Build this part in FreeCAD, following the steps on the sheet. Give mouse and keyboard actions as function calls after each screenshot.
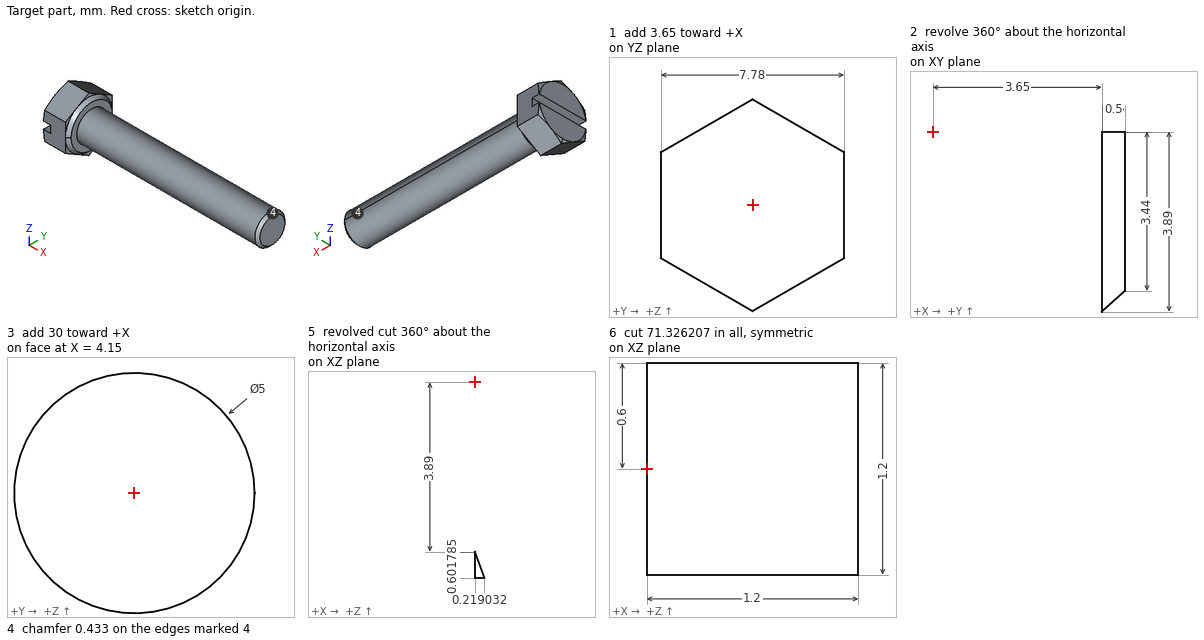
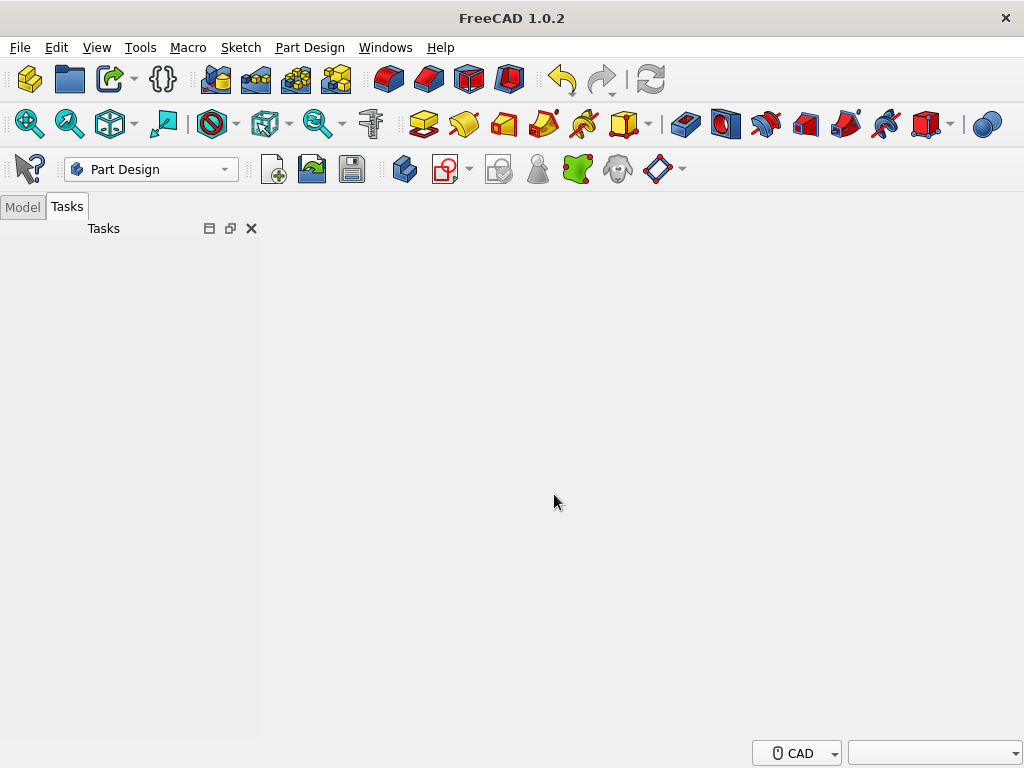
key(ctrl+n)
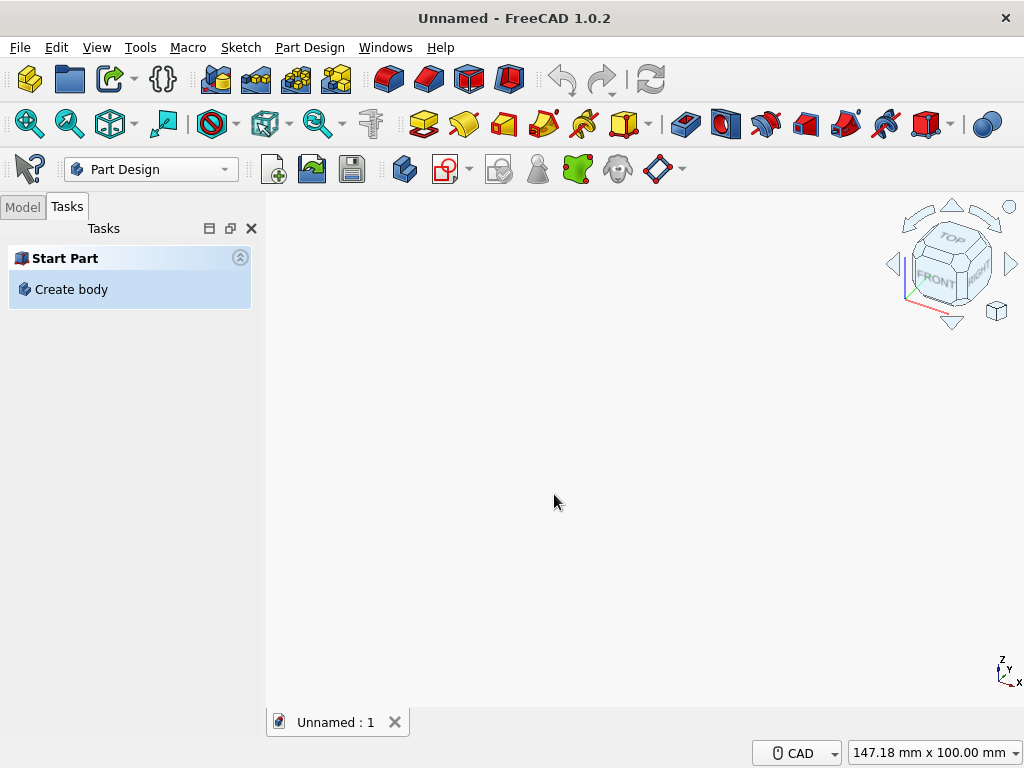
click(446, 170)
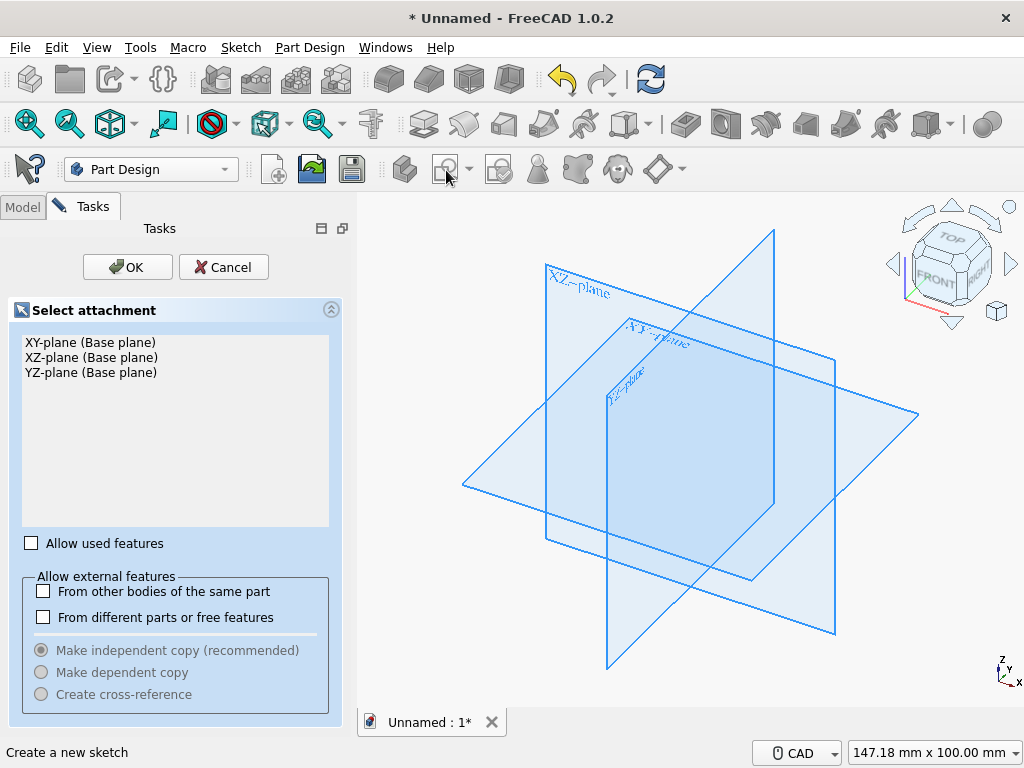
click(82, 372)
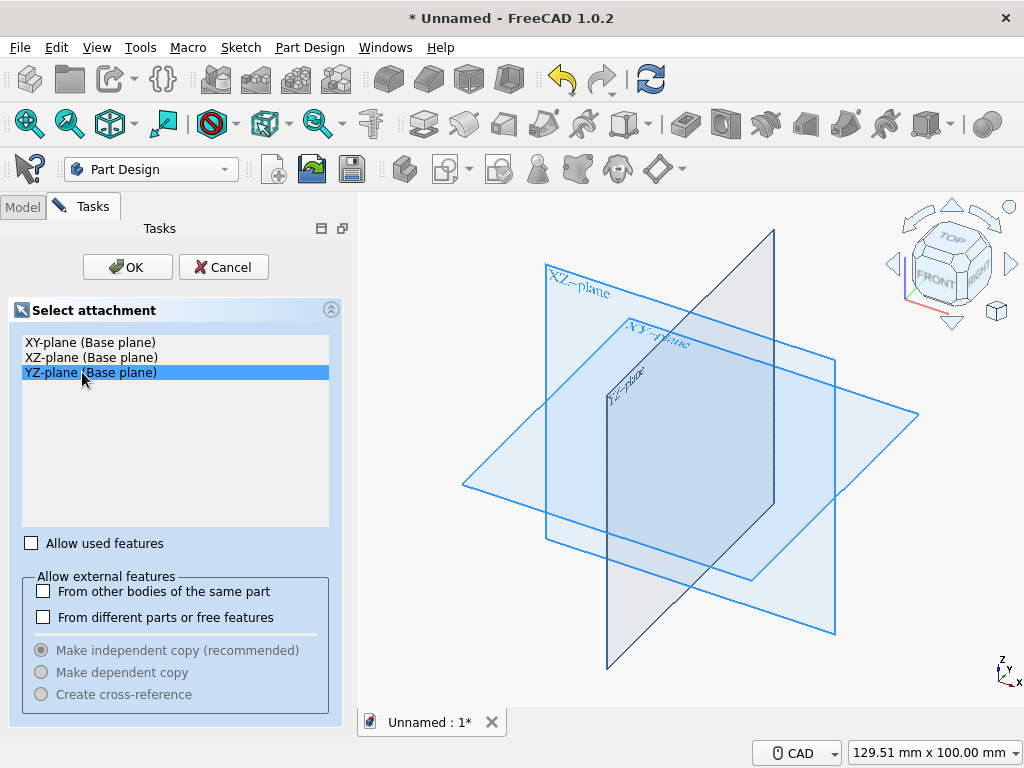
click(128, 267)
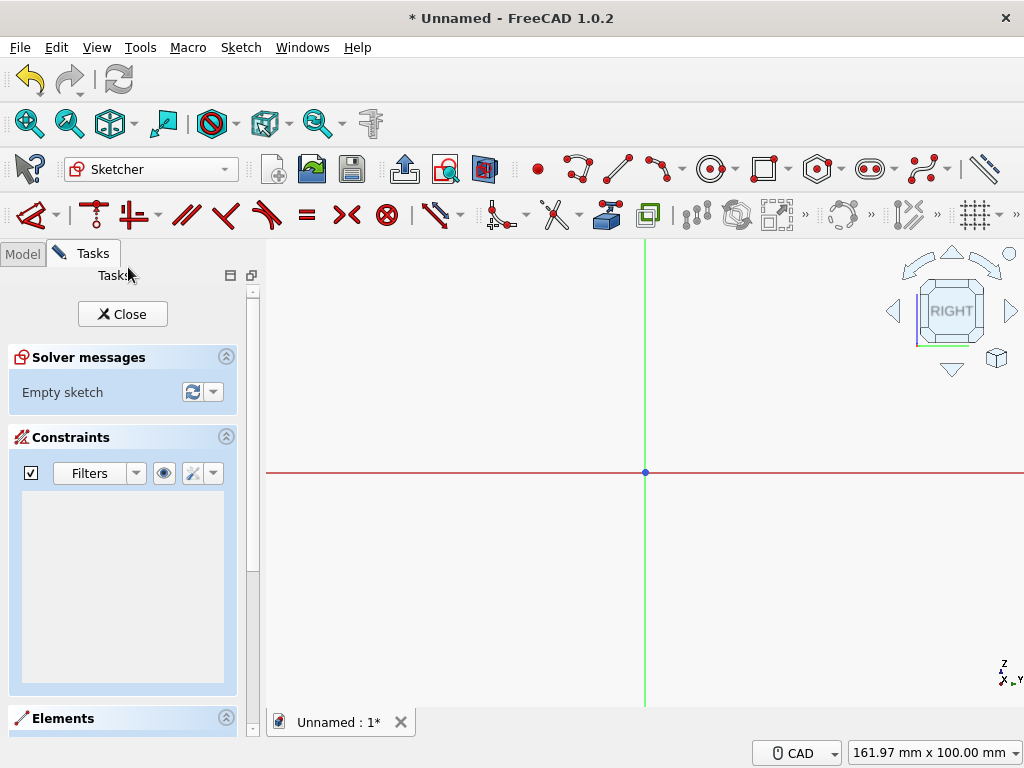
scroll(656, 473, up, 10)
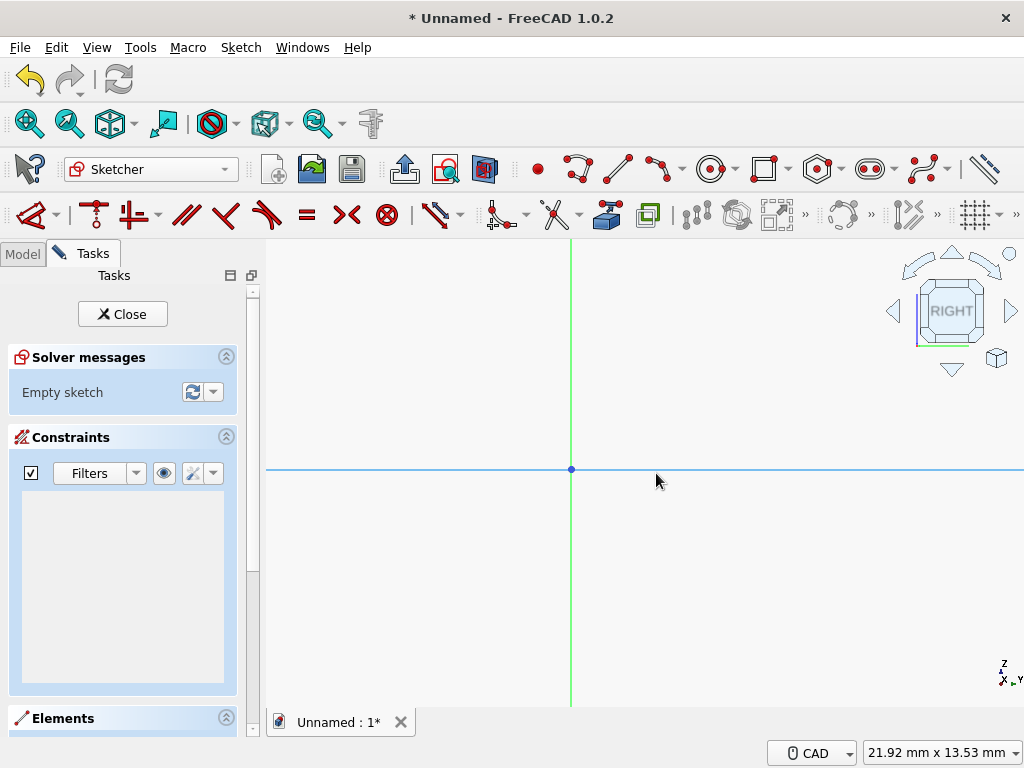
key(g)
key(p)
key(6)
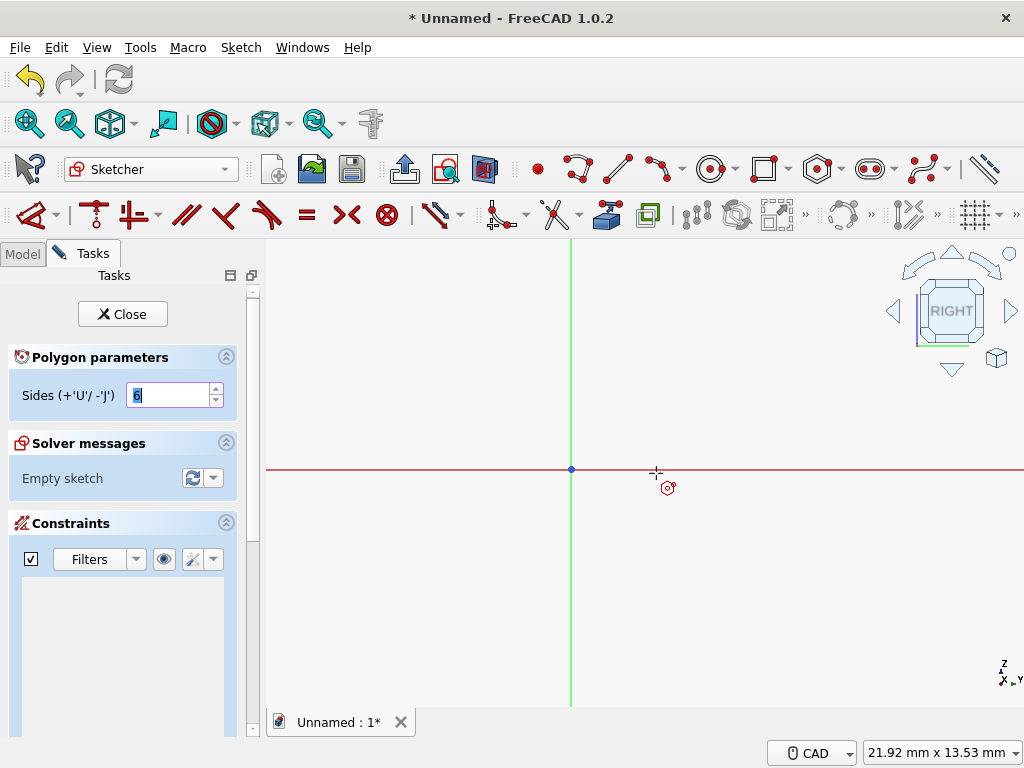
click(571, 470)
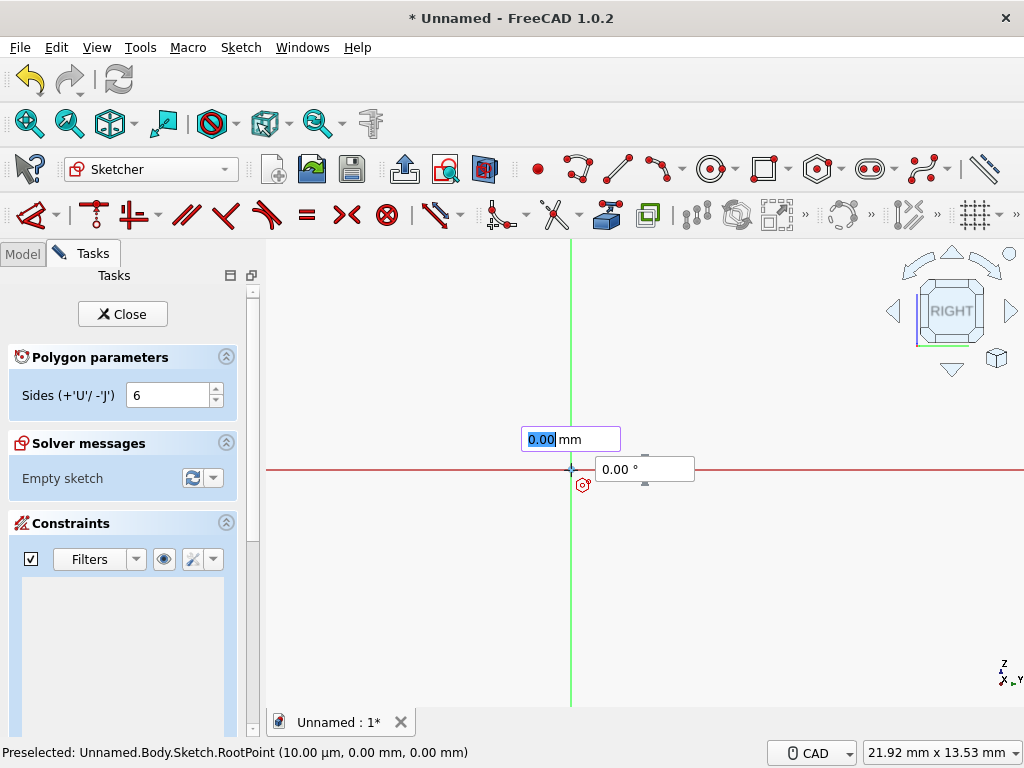
click(571, 625)
right_click(571, 625)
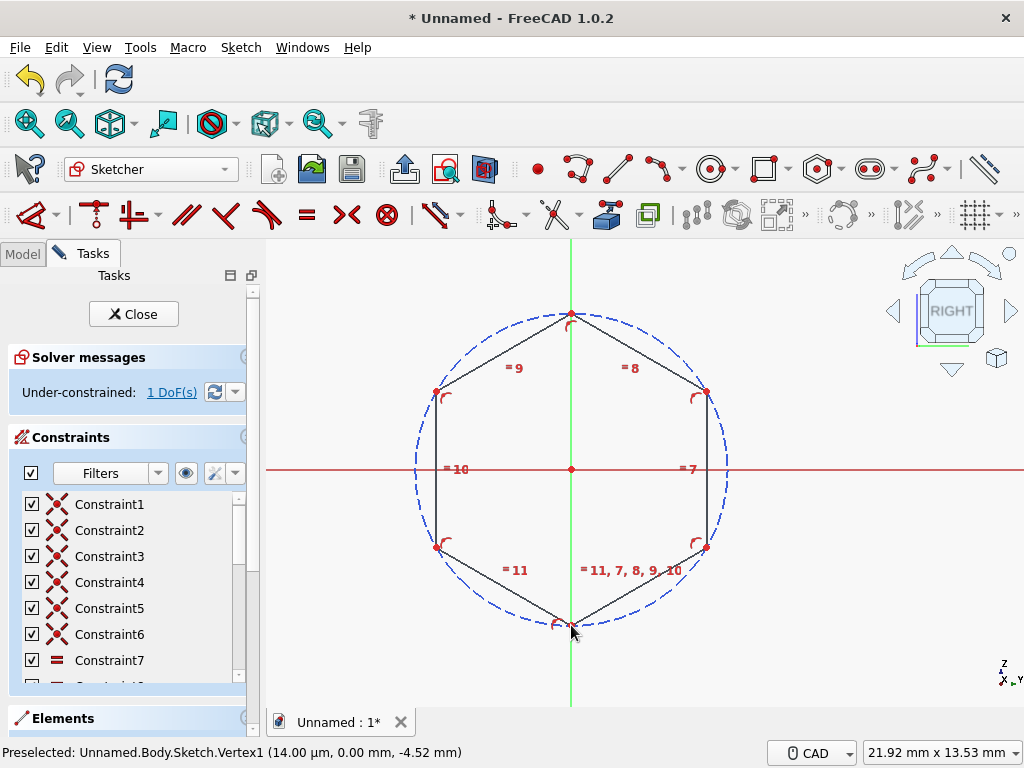
click(436, 392)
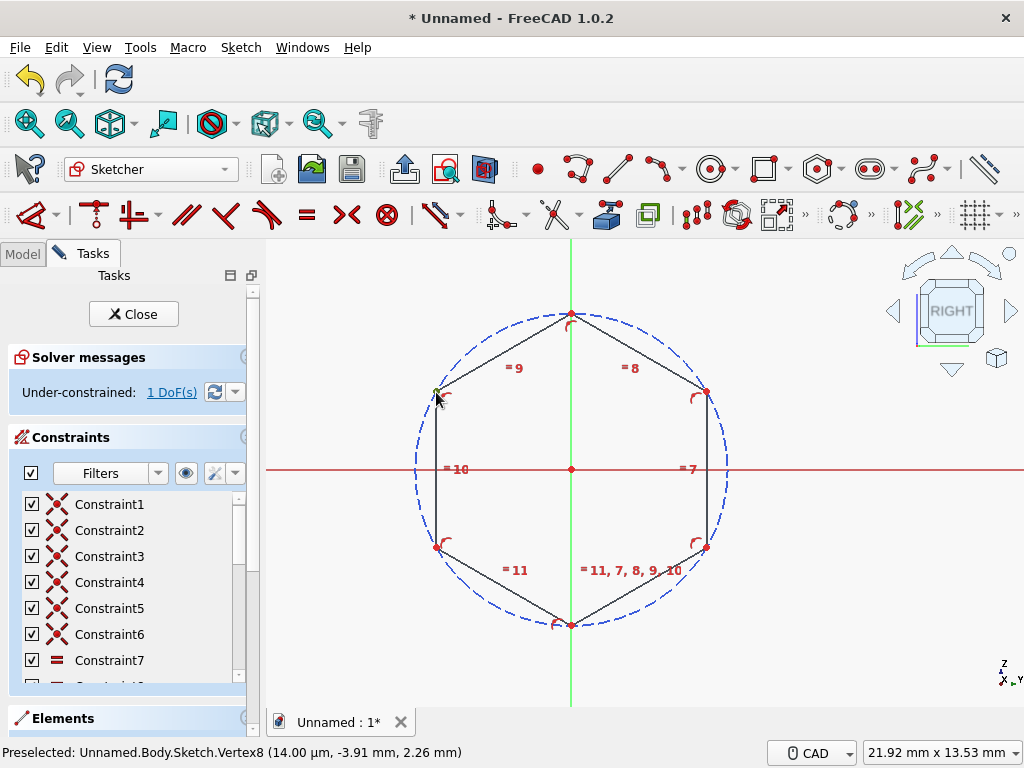
click(707, 548)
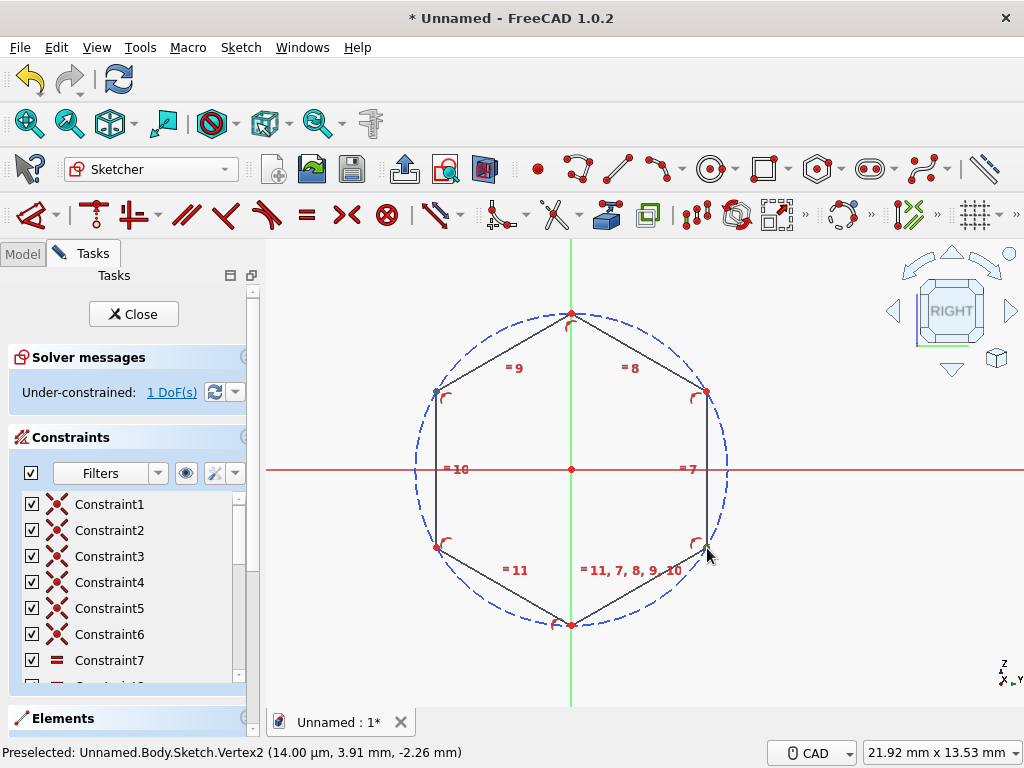
key(l)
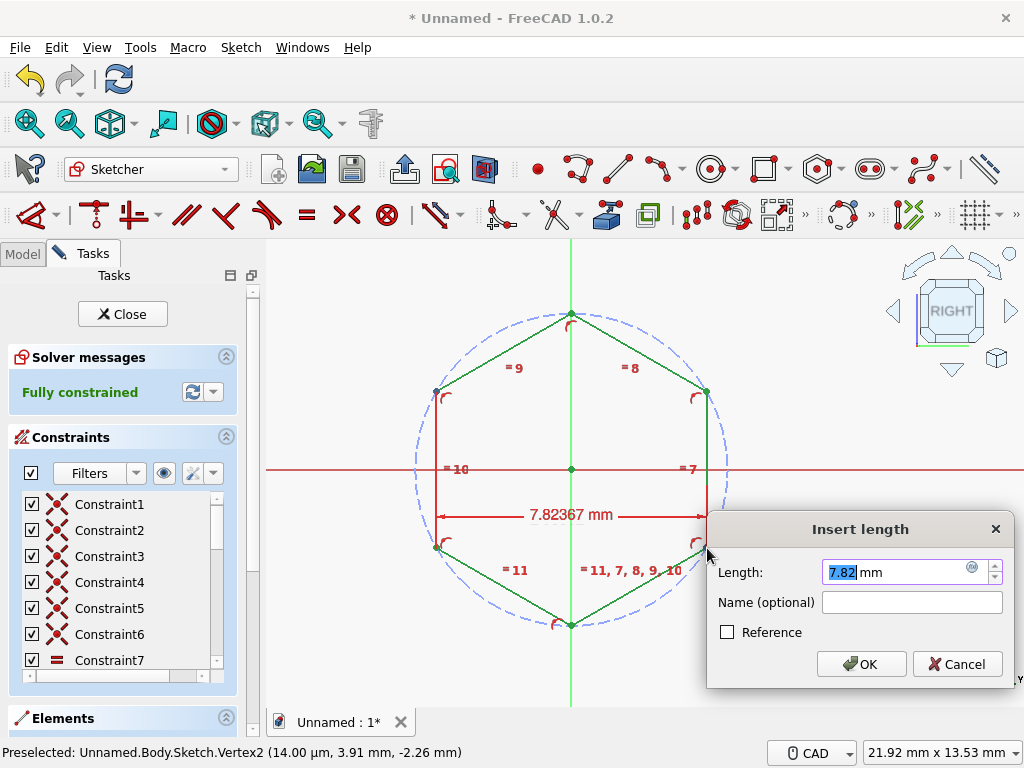
text(7.78)
key(Return)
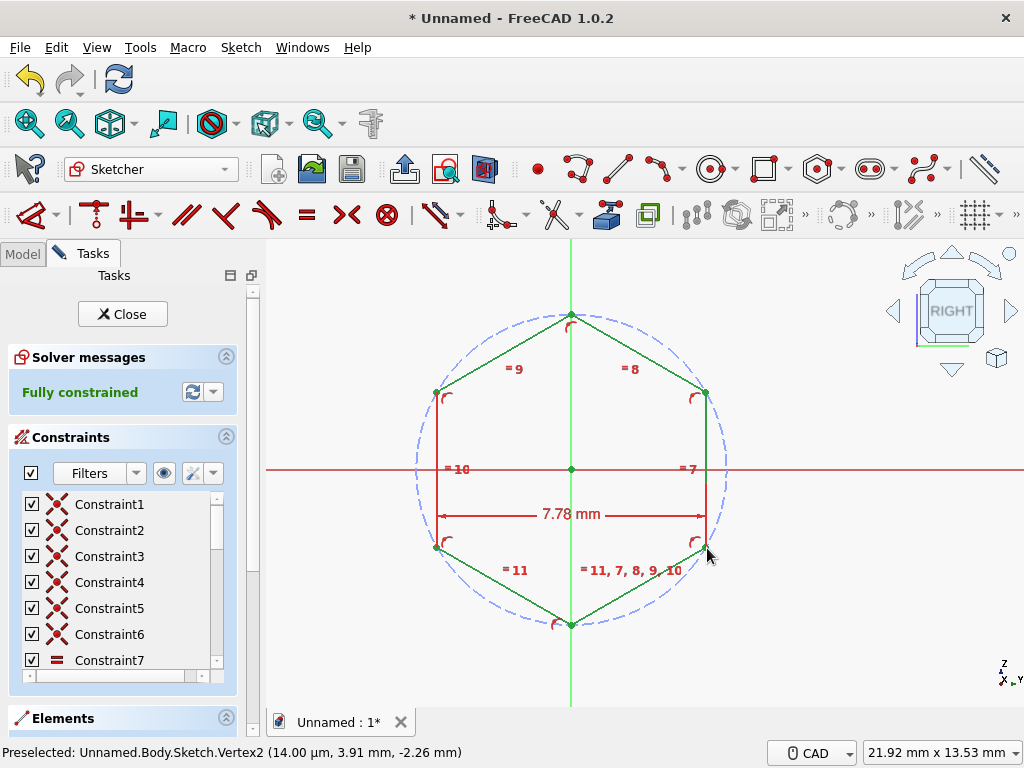
click(123, 314)